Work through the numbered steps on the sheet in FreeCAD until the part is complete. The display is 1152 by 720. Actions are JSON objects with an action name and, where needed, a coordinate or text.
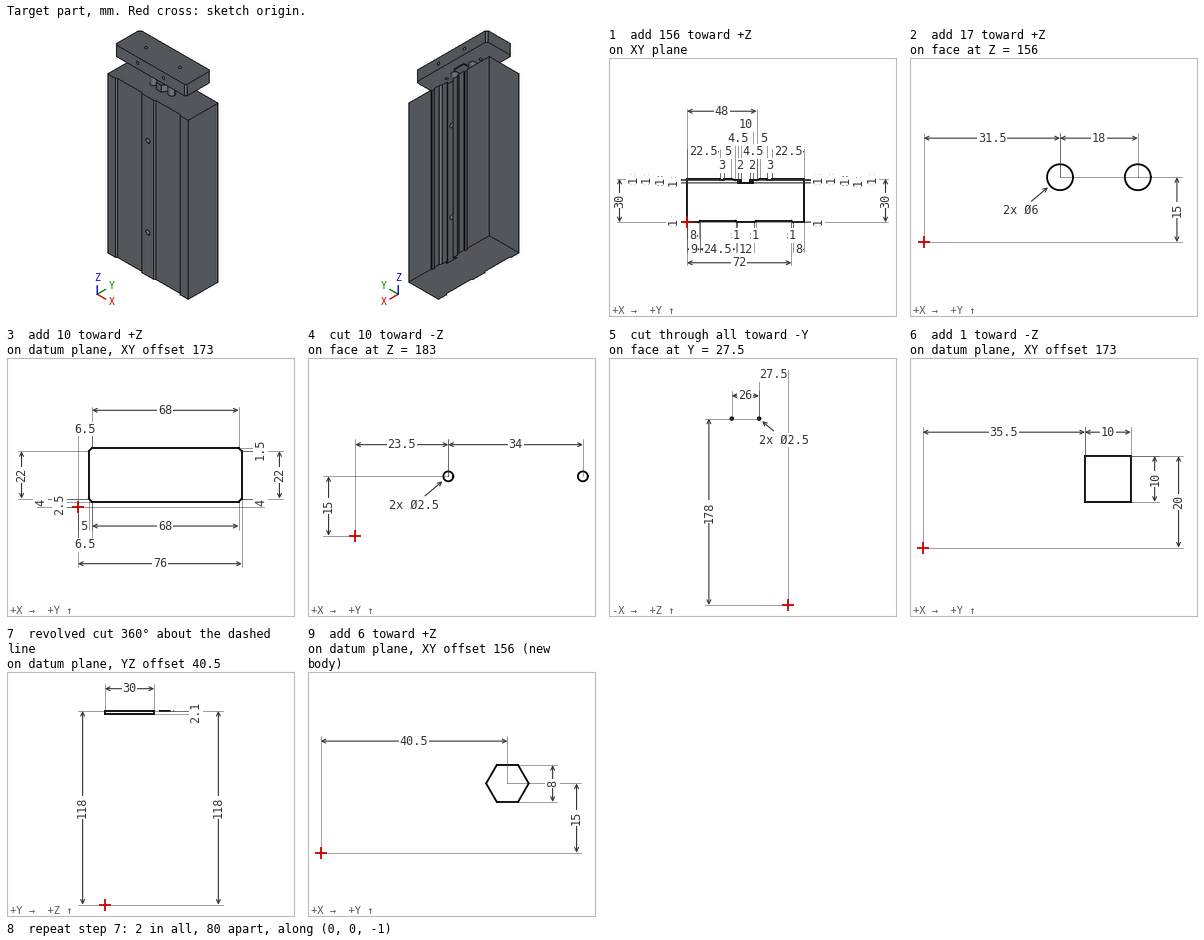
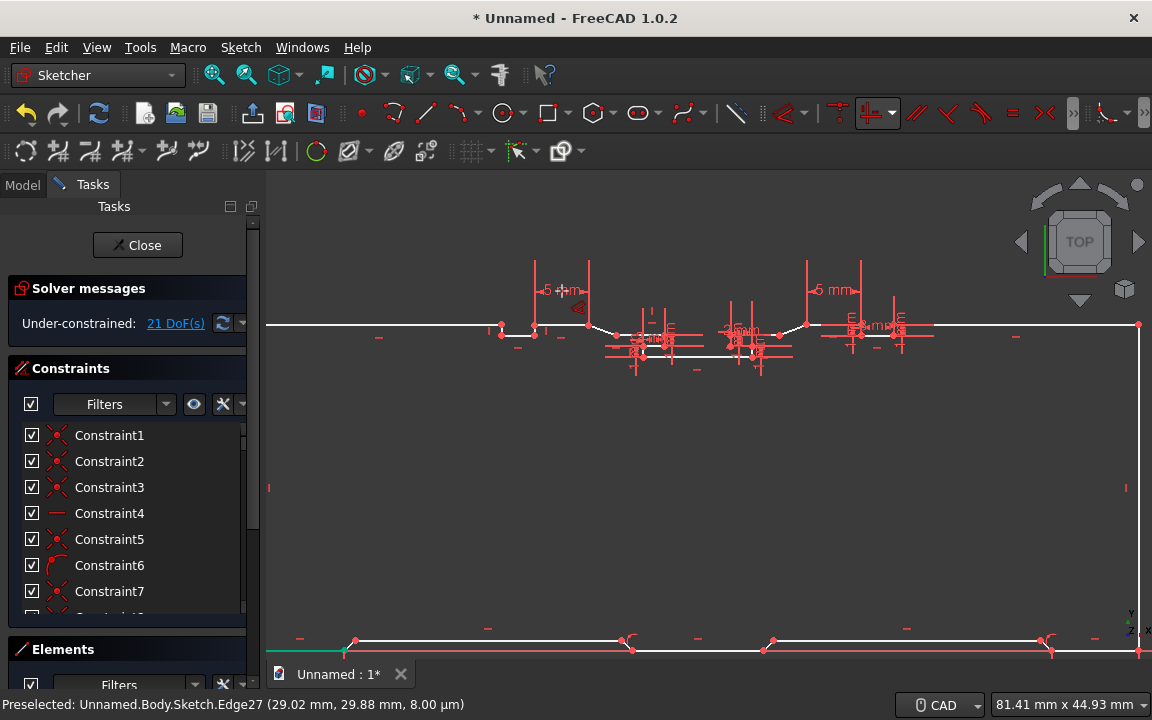
{"action": "scroll", "coordinate": [535, 331], "scroll_direction": "up", "scroll_amount": 7}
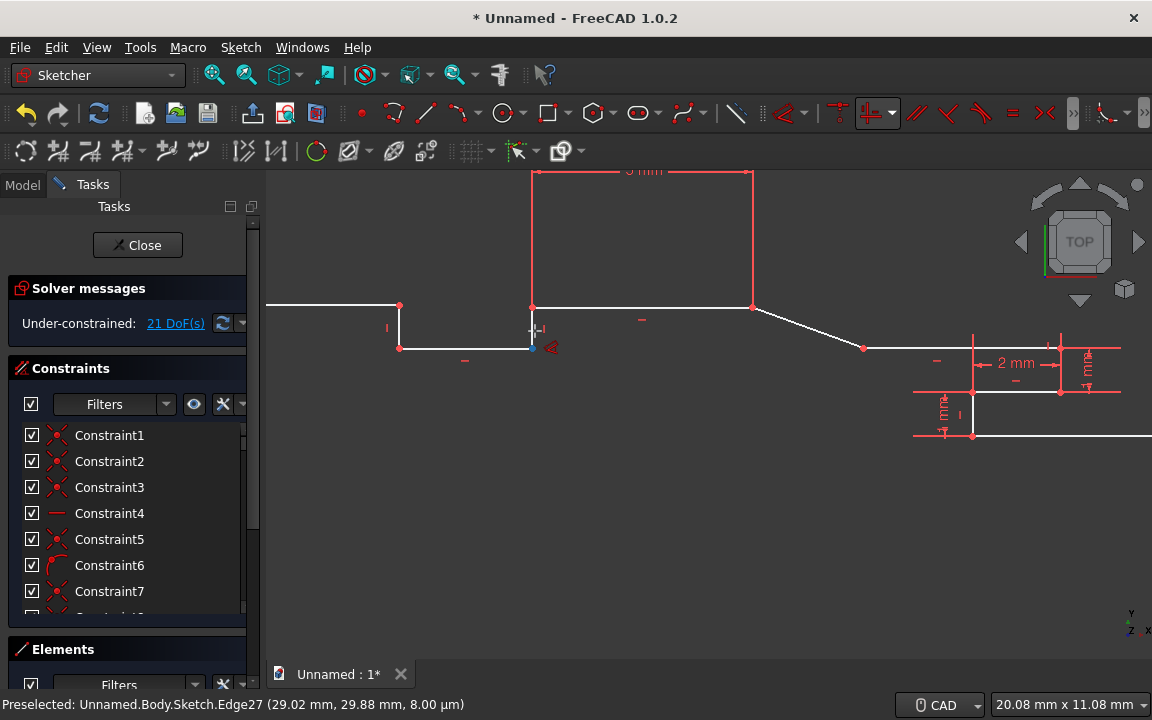
{"action": "left_click", "coordinate": [532, 328]}
{"action": "left_click", "coordinate": [498, 328]}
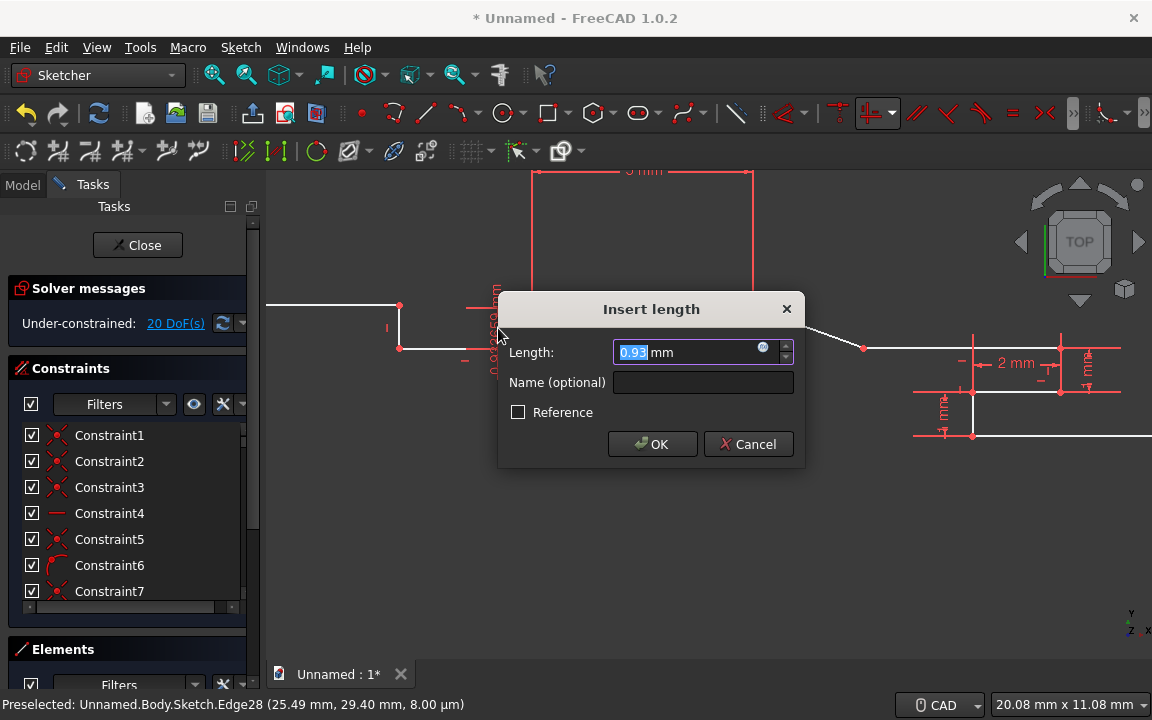
{"action": "type", "text": "1"}
{"action": "key", "text": "Return"}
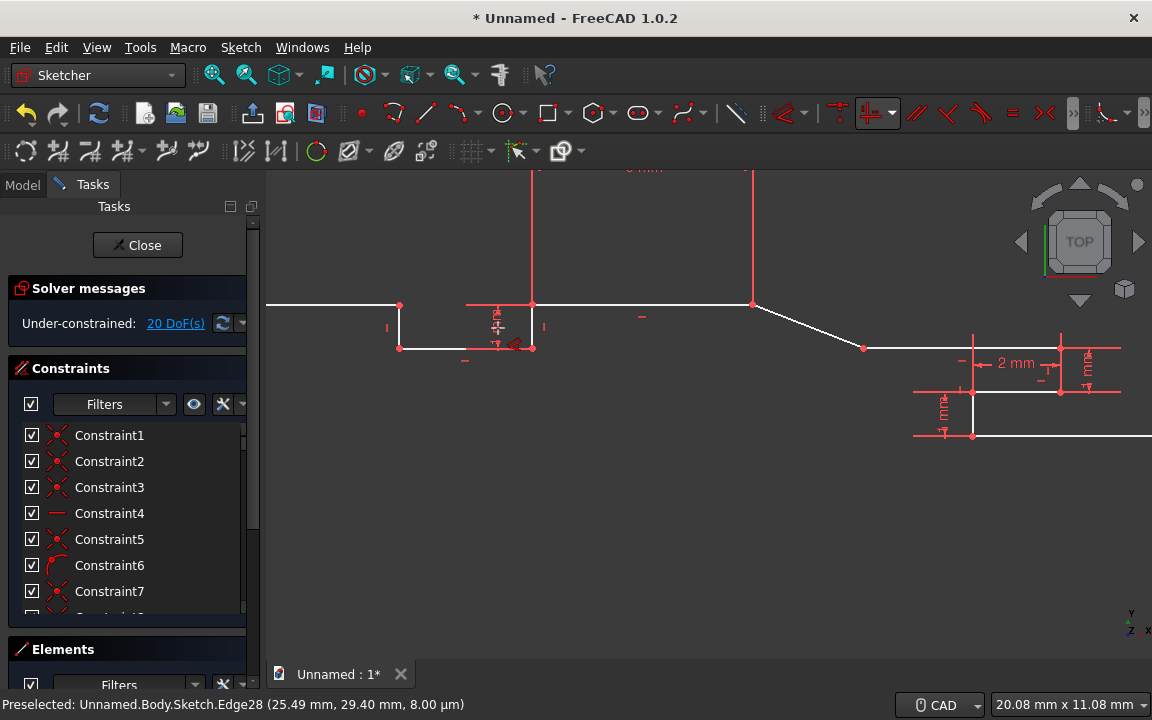
{"action": "scroll", "coordinate": [554, 328], "scroll_direction": "down", "scroll_amount": 10}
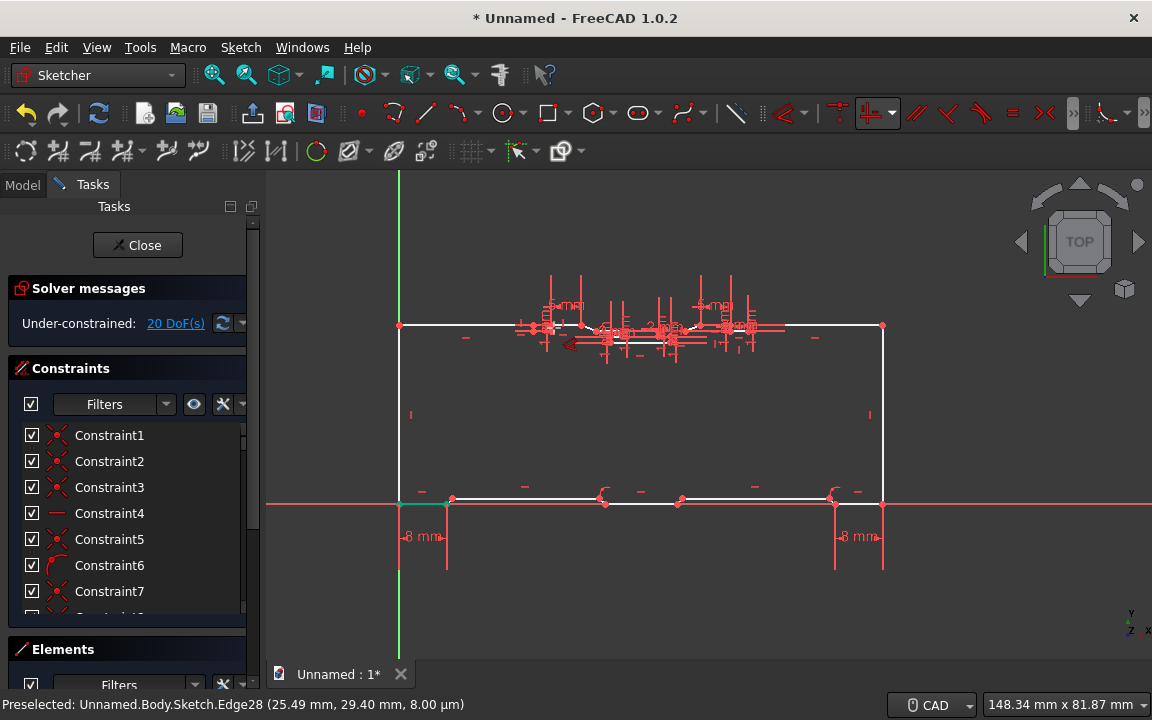
{"action": "scroll", "coordinate": [546, 331], "scroll_direction": "up", "scroll_amount": 5}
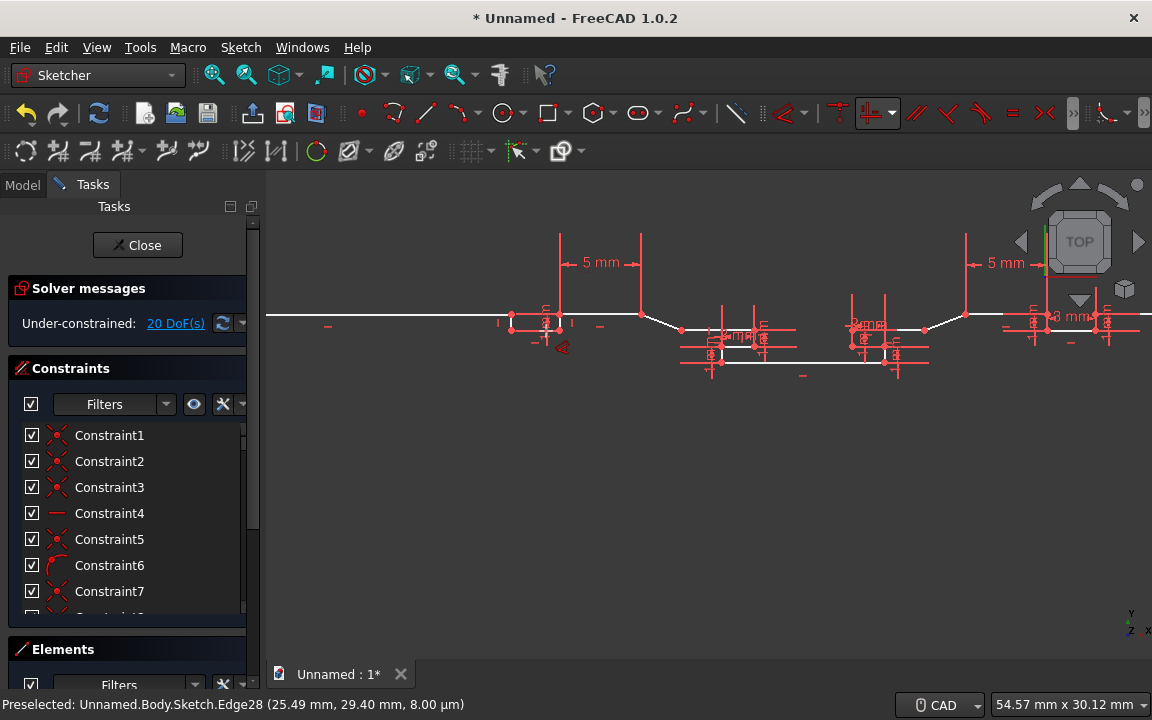
{"action": "left_click", "coordinate": [545, 331]}
{"action": "left_click", "coordinate": [535, 297]}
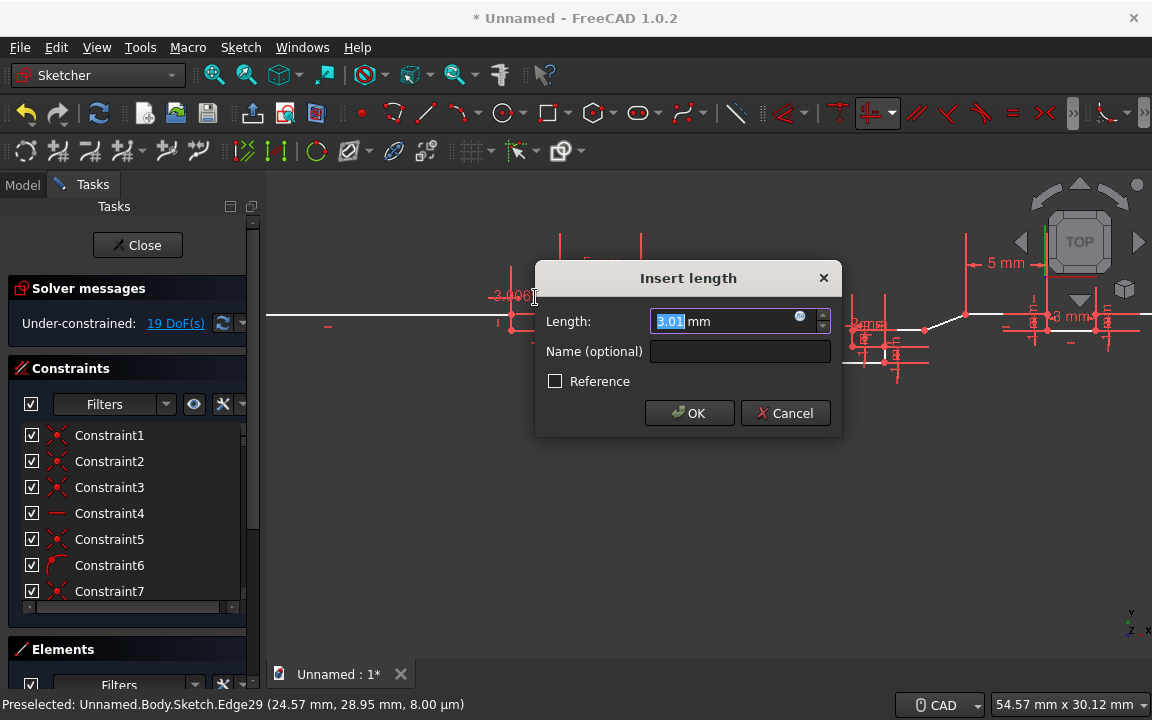
{"action": "type", "text": "3"}
{"action": "key", "text": "Return"}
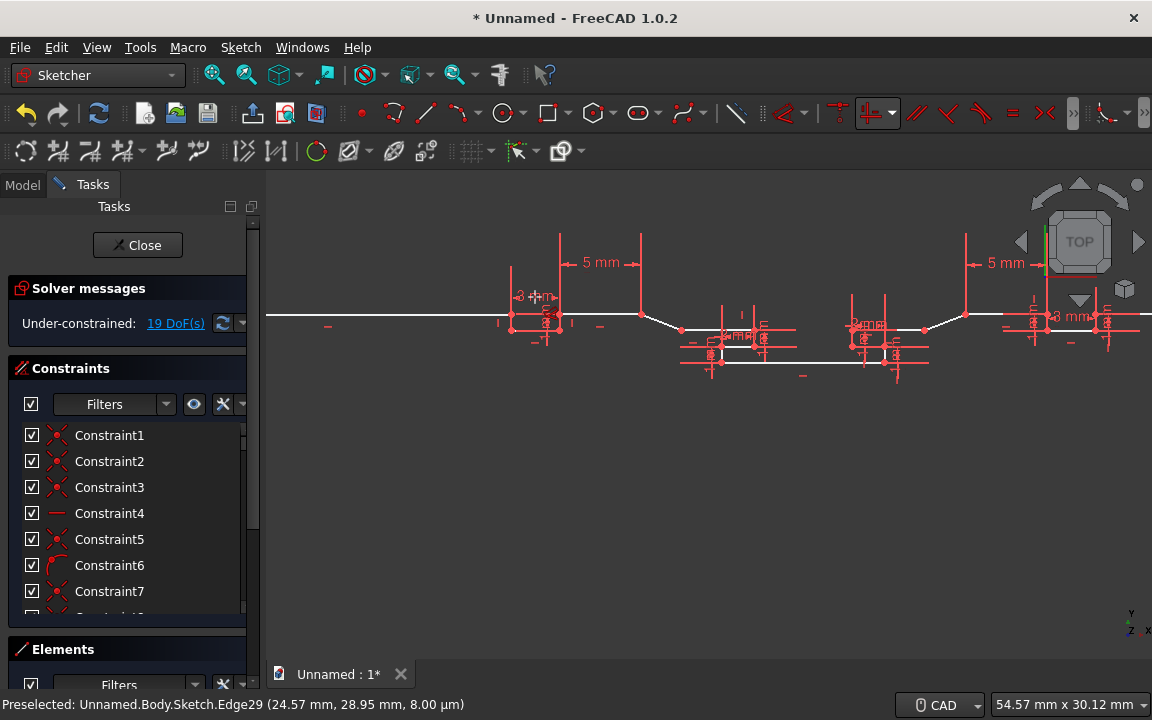
{"action": "scroll", "coordinate": [511, 323], "scroll_direction": "up", "scroll_amount": 5}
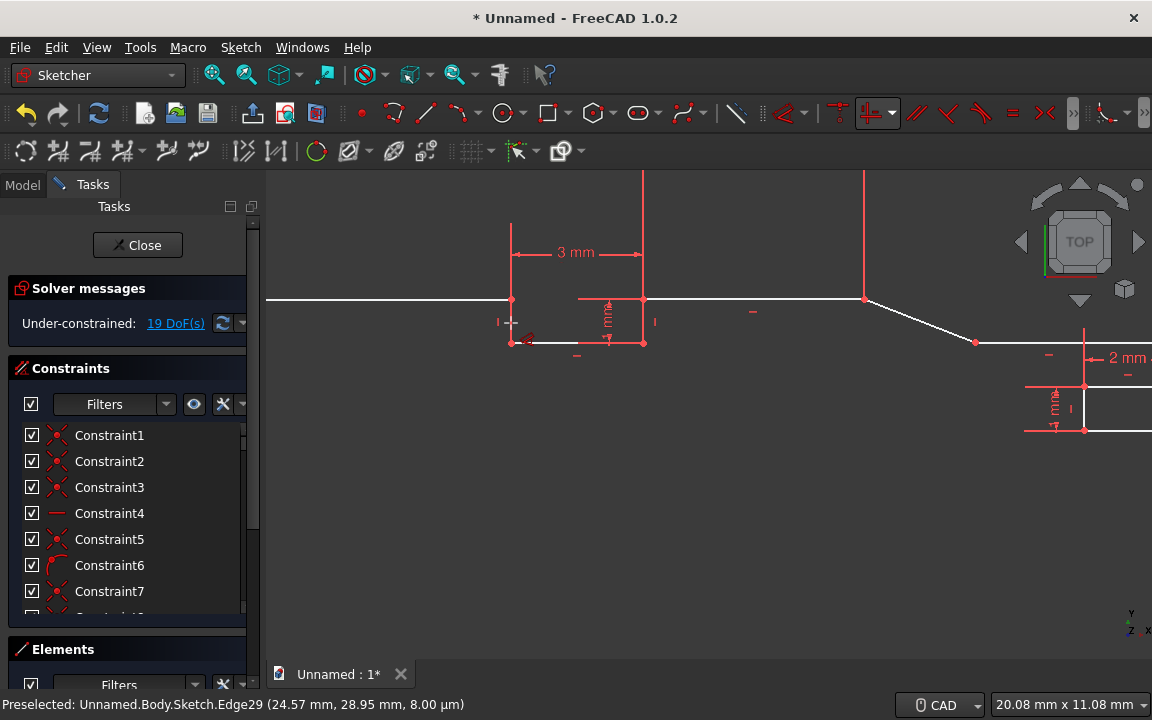
{"action": "left_click", "coordinate": [511, 322]}
{"action": "left_click", "coordinate": [477, 322]}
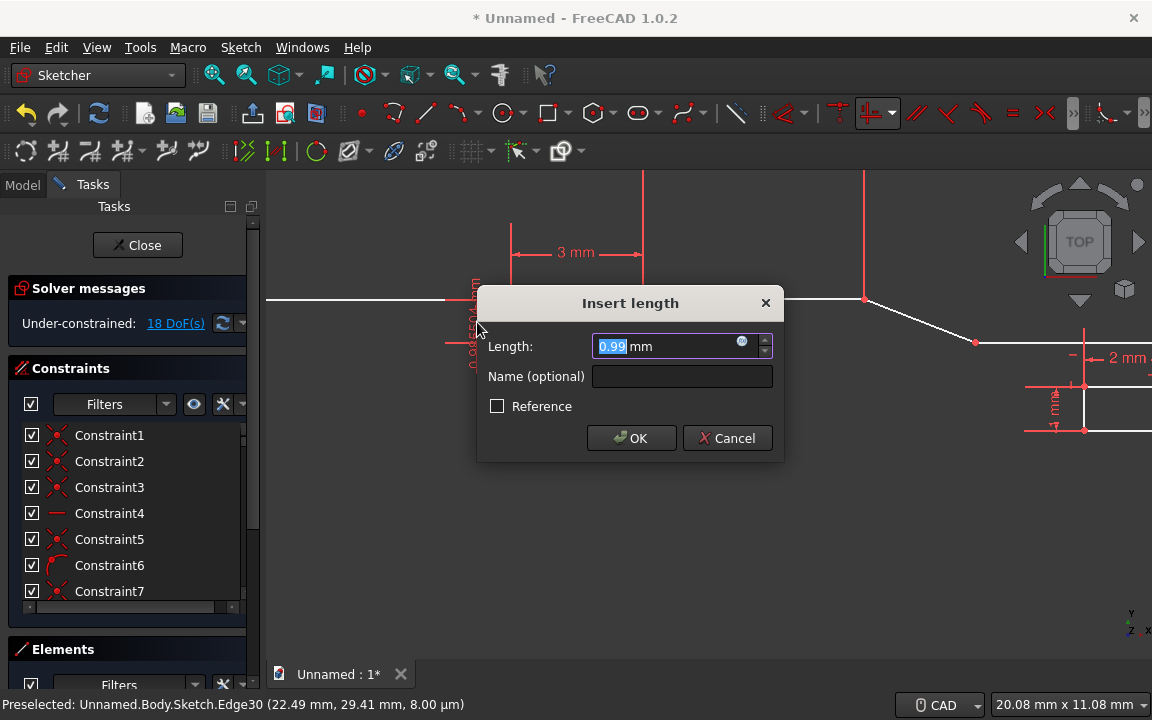
{"action": "type", "text": "1"}
{"action": "key", "text": "Return"}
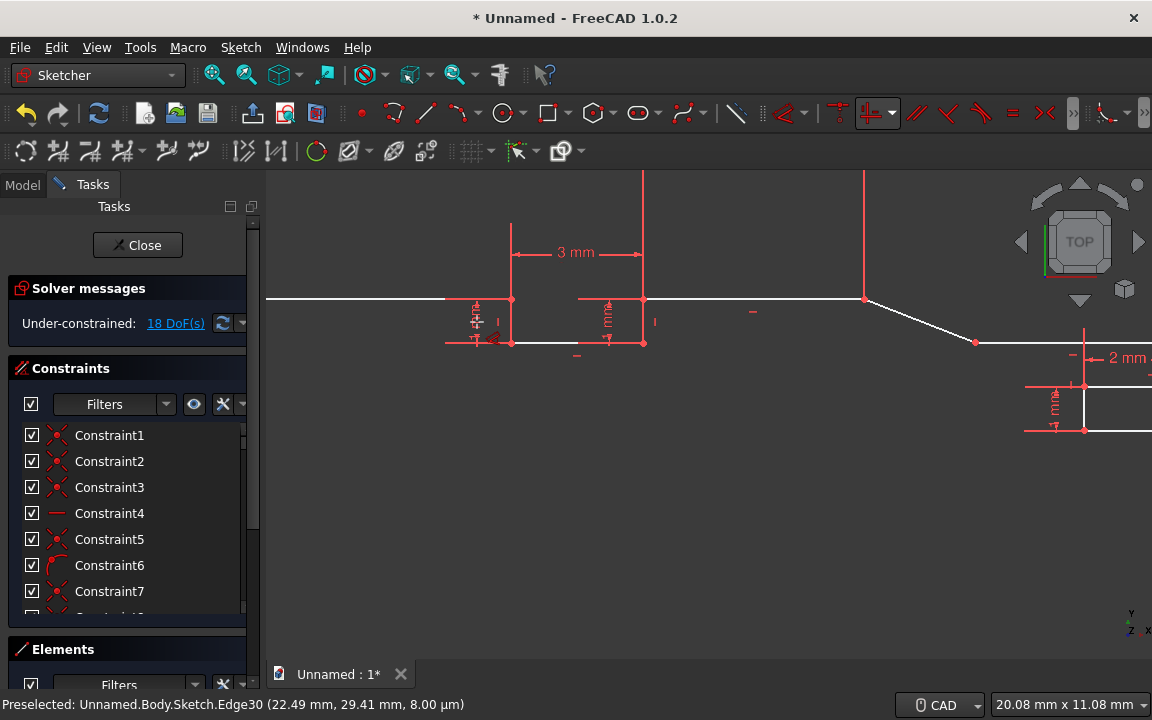
{"action": "scroll", "coordinate": [536, 329], "scroll_direction": "down", "scroll_amount": 10}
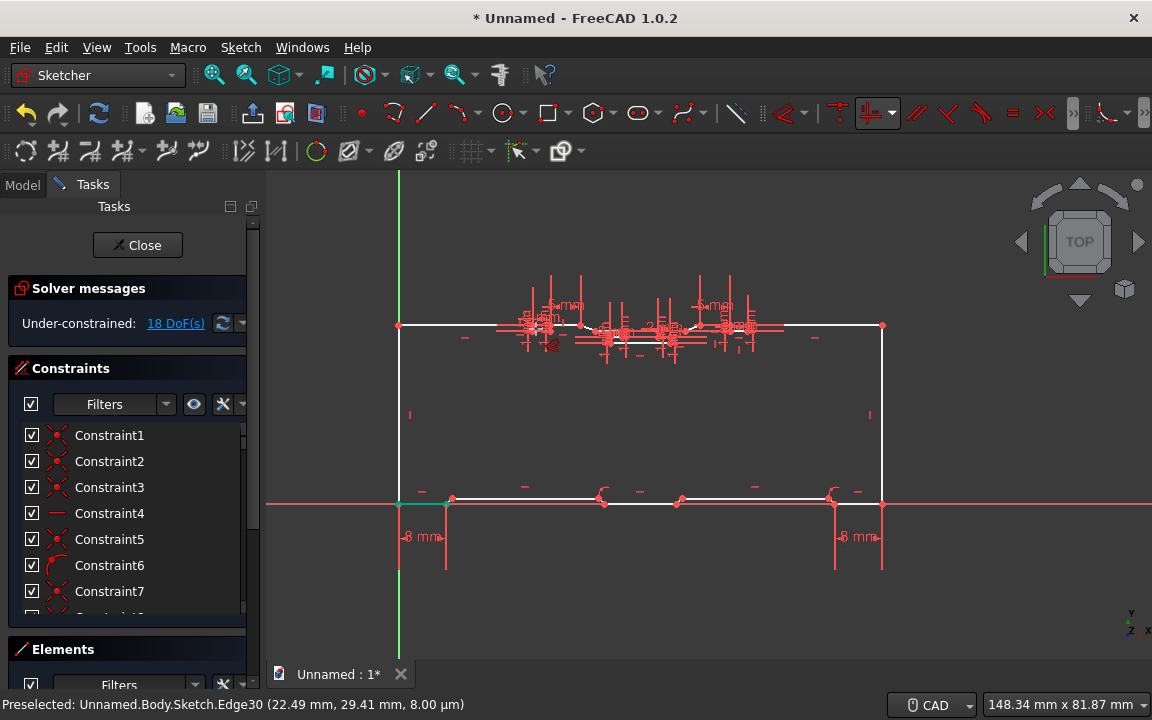
{"action": "left_click", "coordinate": [626, 504]}
{"action": "left_click", "coordinate": [641, 538]}